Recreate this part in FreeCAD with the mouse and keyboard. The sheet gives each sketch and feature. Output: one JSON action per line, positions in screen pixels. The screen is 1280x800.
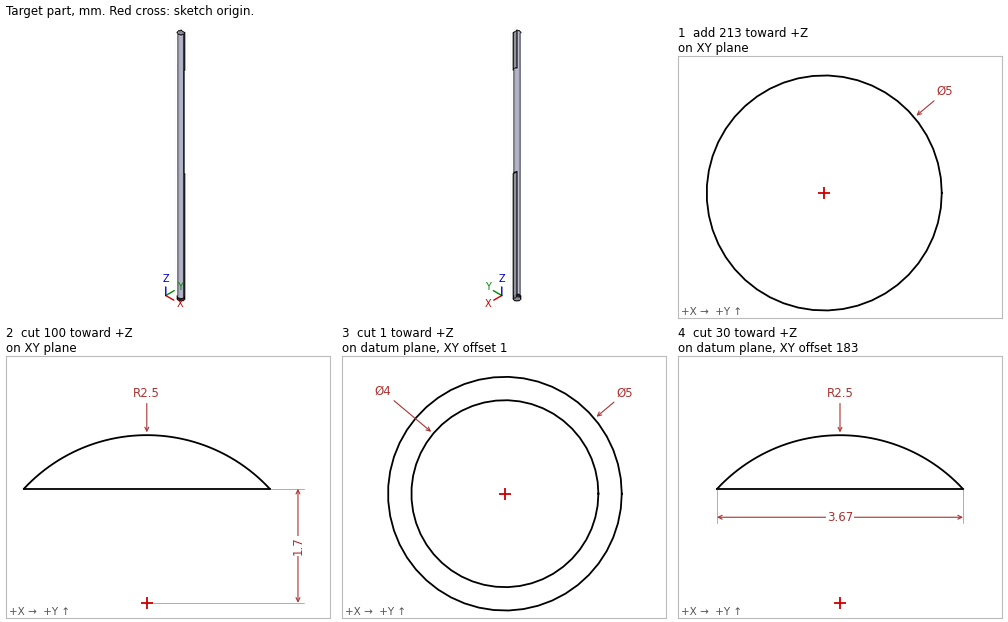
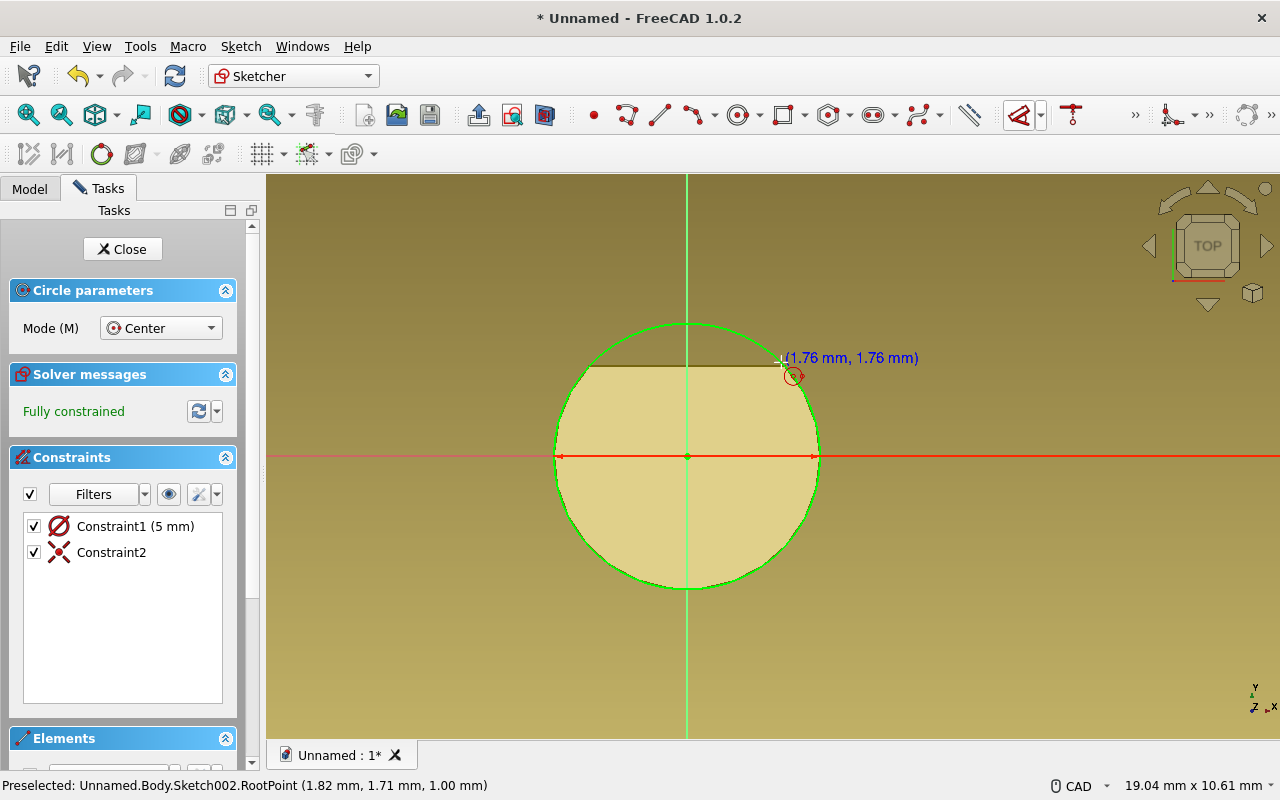
{"action": "left_click", "coordinate": [687, 456]}
{"action": "mouse_move", "coordinate": [762, 381]}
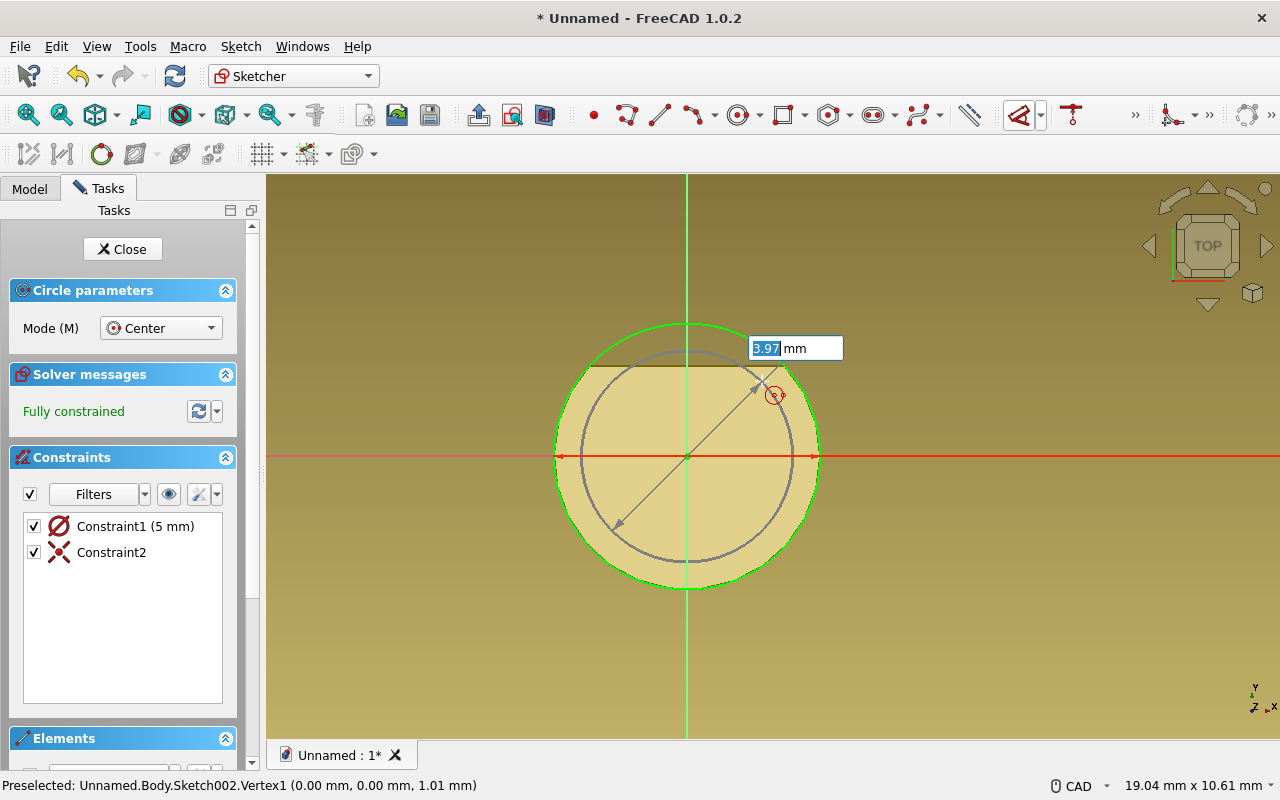
{"action": "type", "text": "4"}
{"action": "key", "text": "Return"}
{"action": "key", "text": "Escape"}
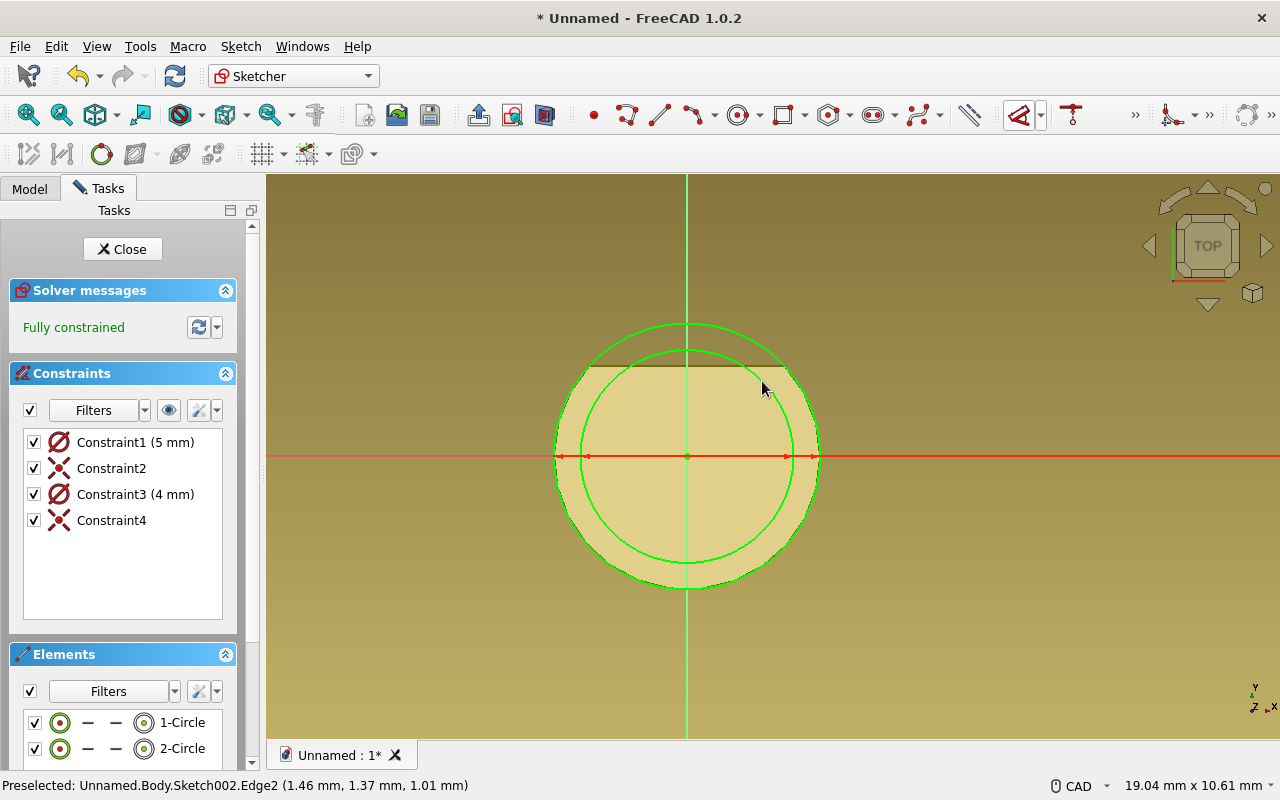
{"action": "left_click", "coordinate": [123, 249]}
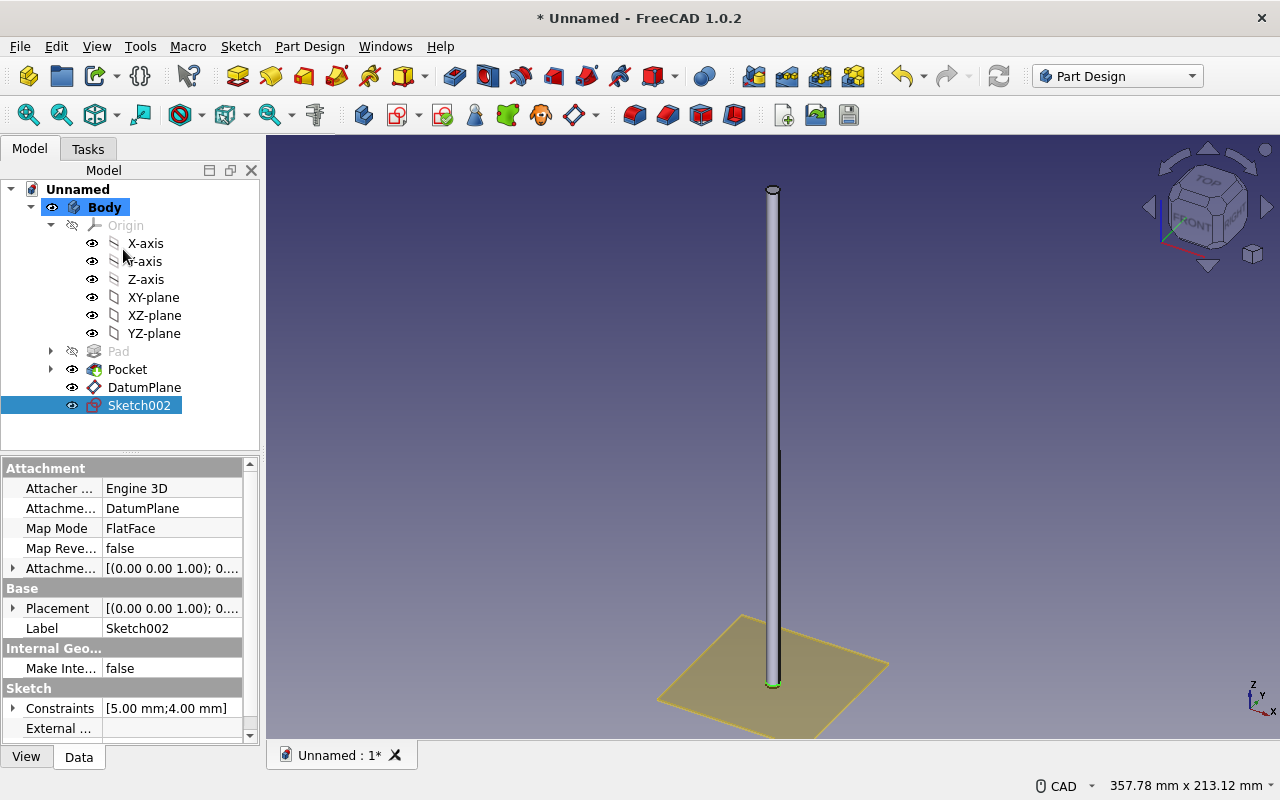
{"action": "left_click", "coordinate": [455, 76]}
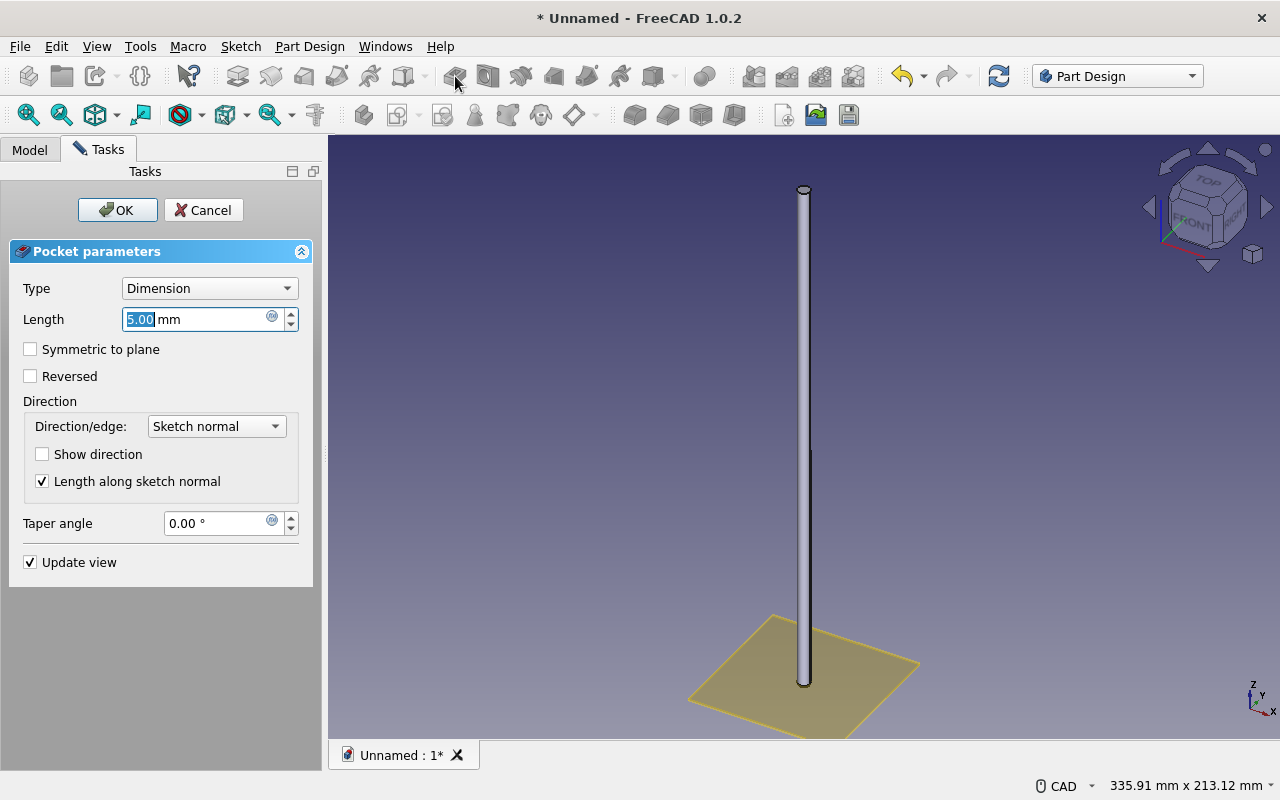
{"action": "type", "text": "1"}
{"action": "key", "text": "Tab"}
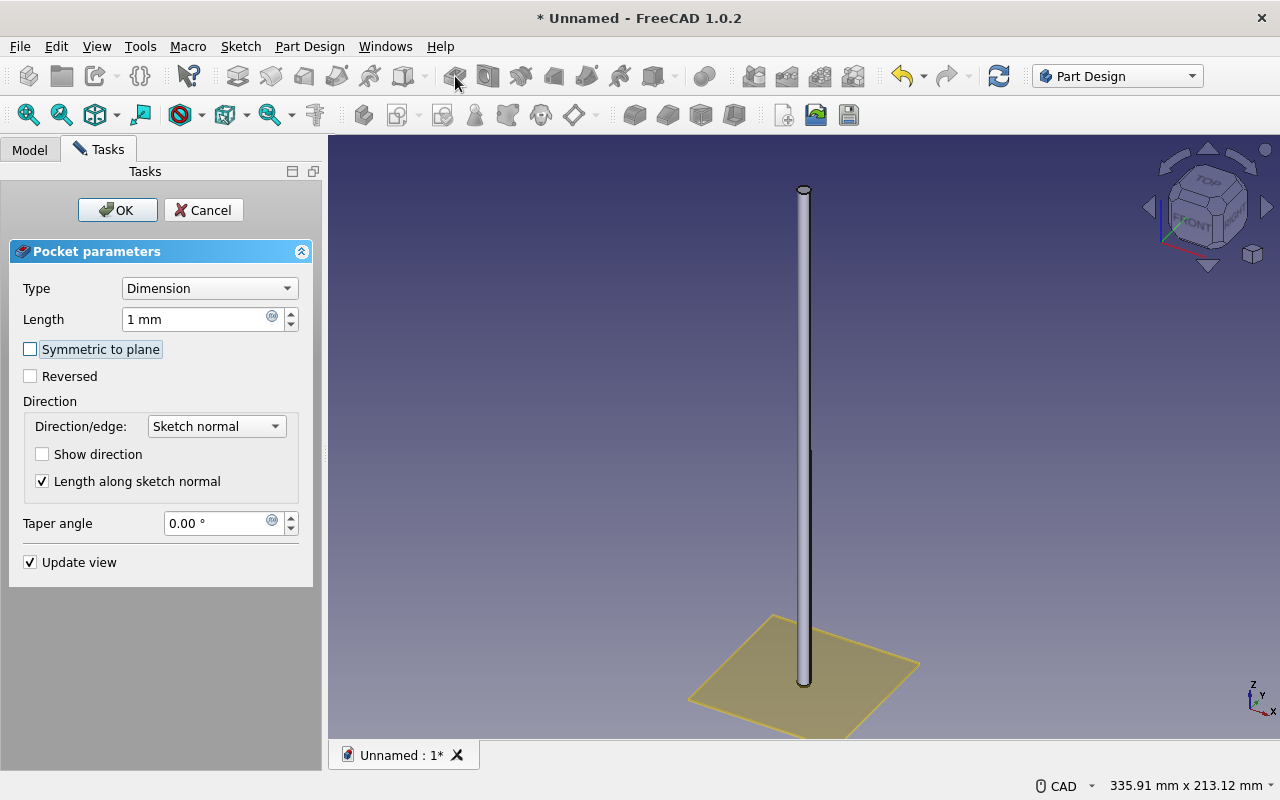
{"action": "left_click", "coordinate": [31, 376]}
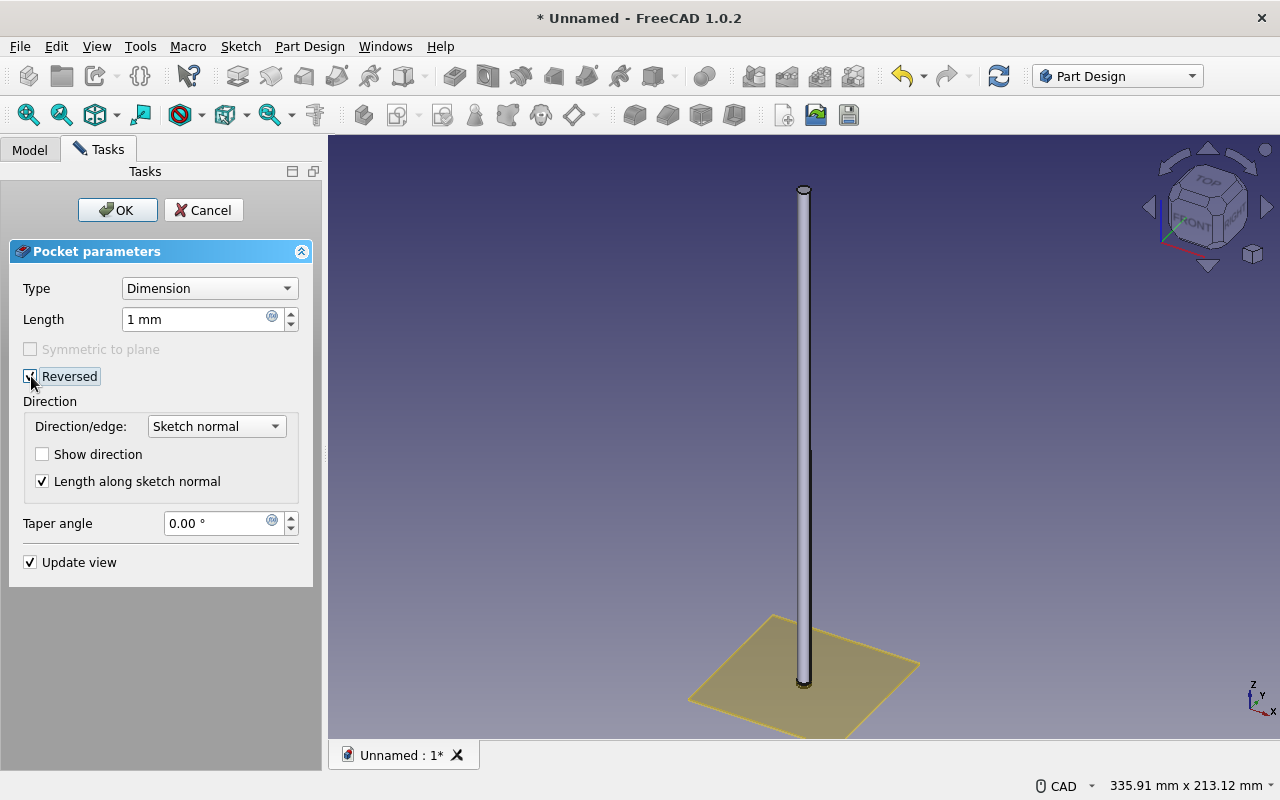
{"action": "left_click", "coordinate": [118, 210]}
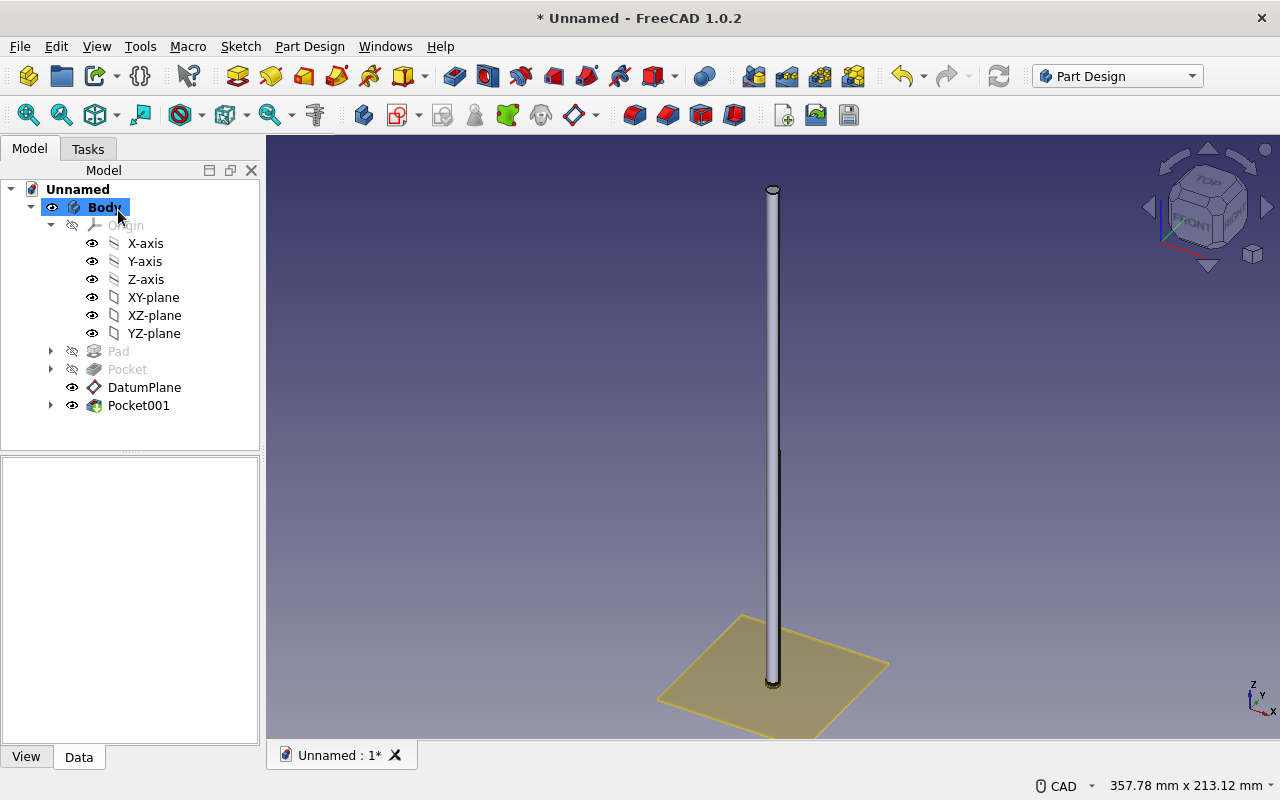
{"action": "left_click", "coordinate": [117, 387]}
{"action": "key", "text": "space"}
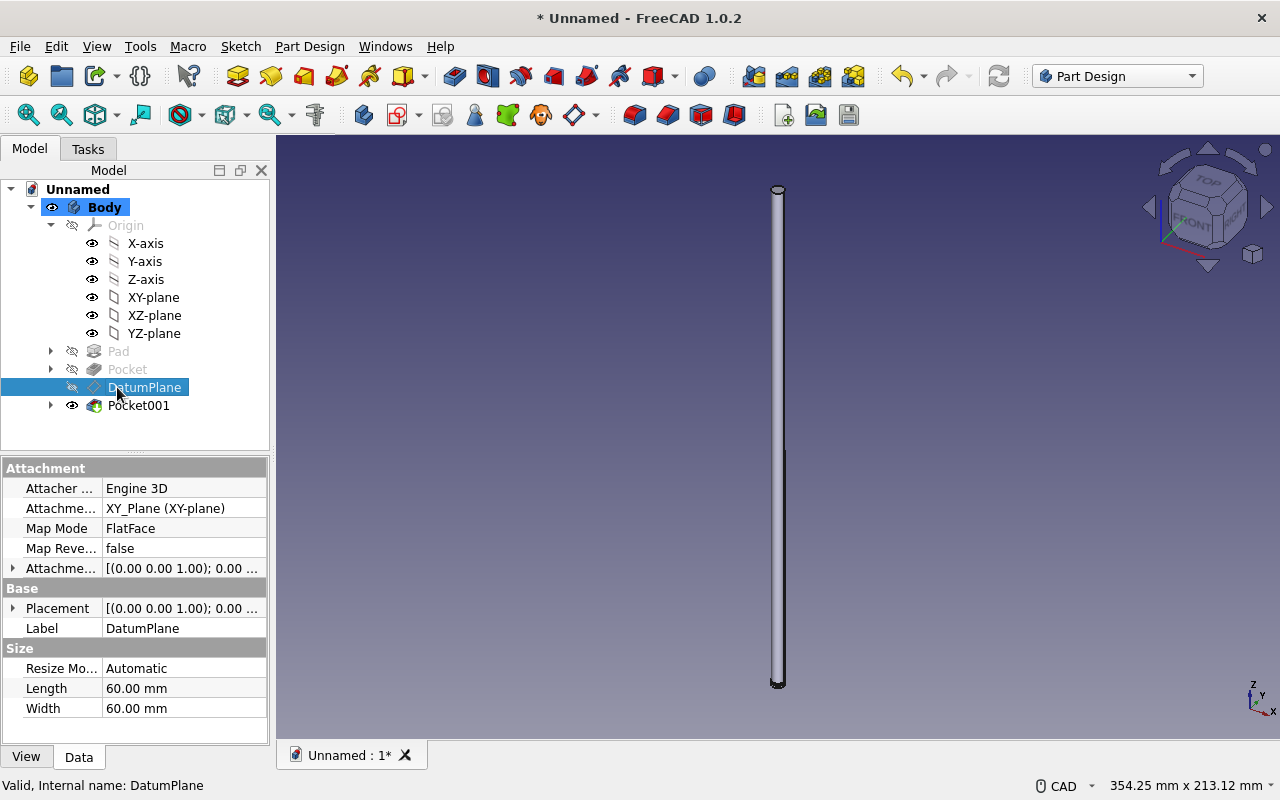
{"action": "left_click", "coordinate": [137, 297]}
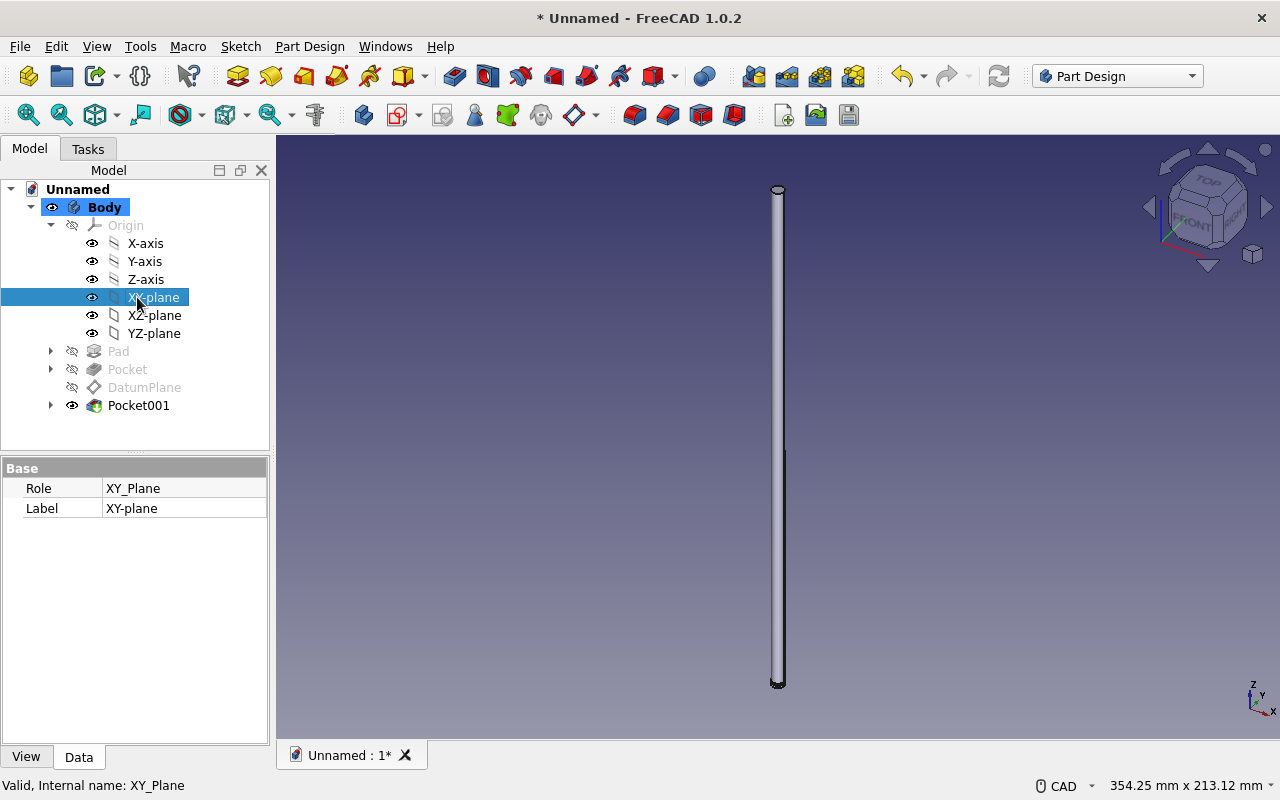
{"action": "left_click", "coordinate": [574, 116]}